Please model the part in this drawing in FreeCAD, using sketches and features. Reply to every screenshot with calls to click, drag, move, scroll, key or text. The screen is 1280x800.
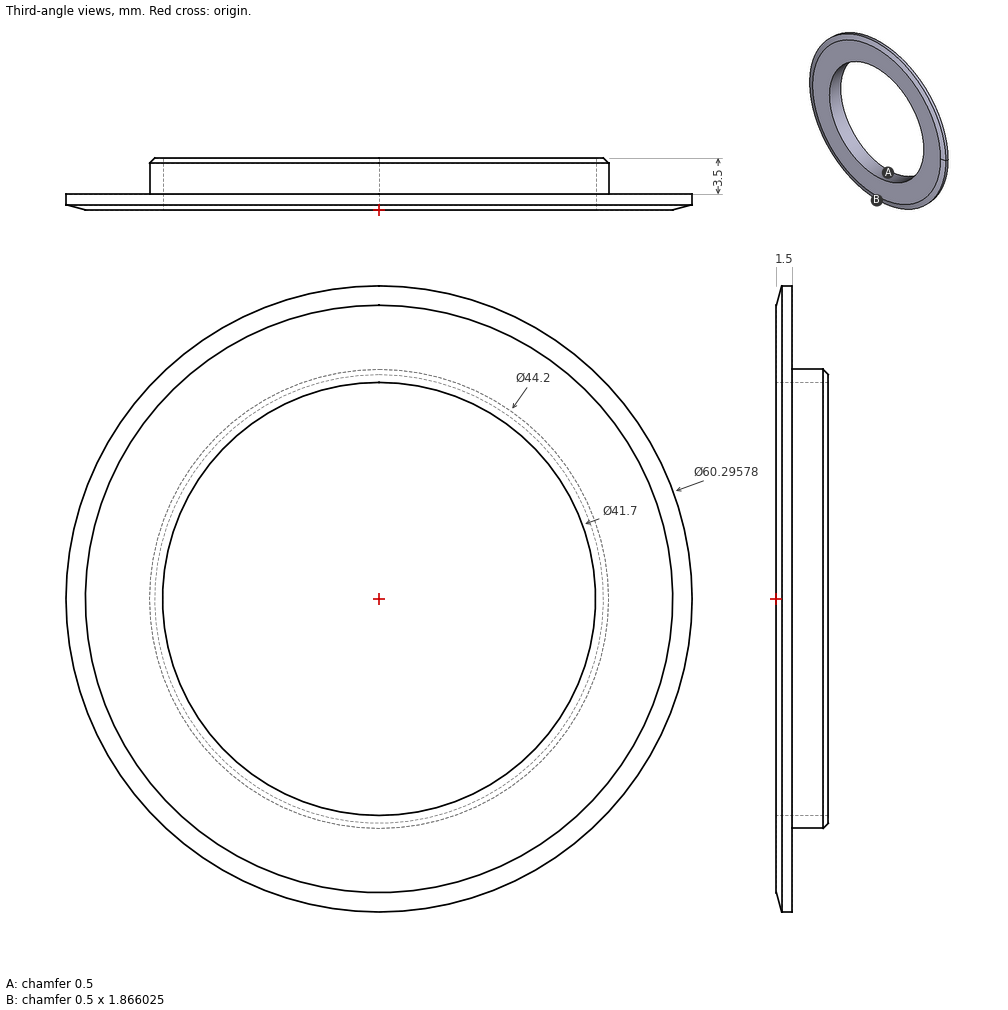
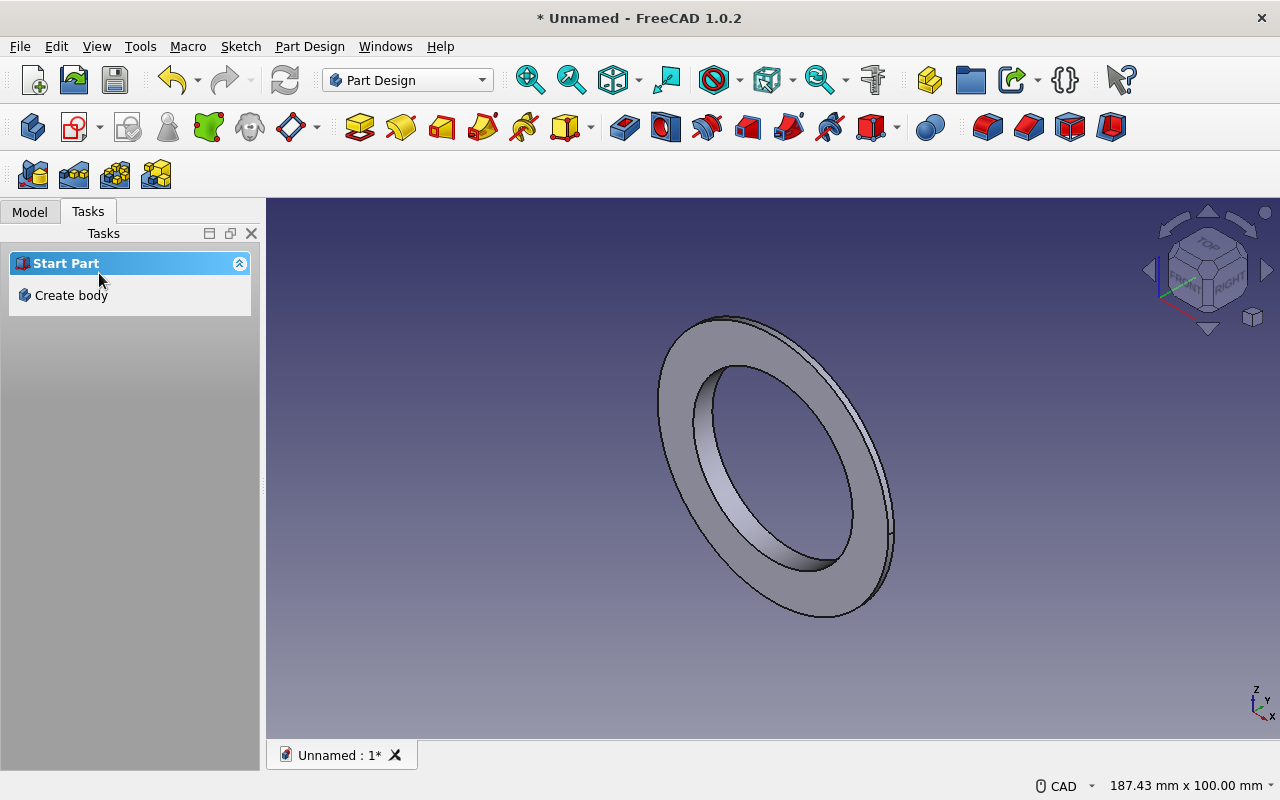
click(737, 320)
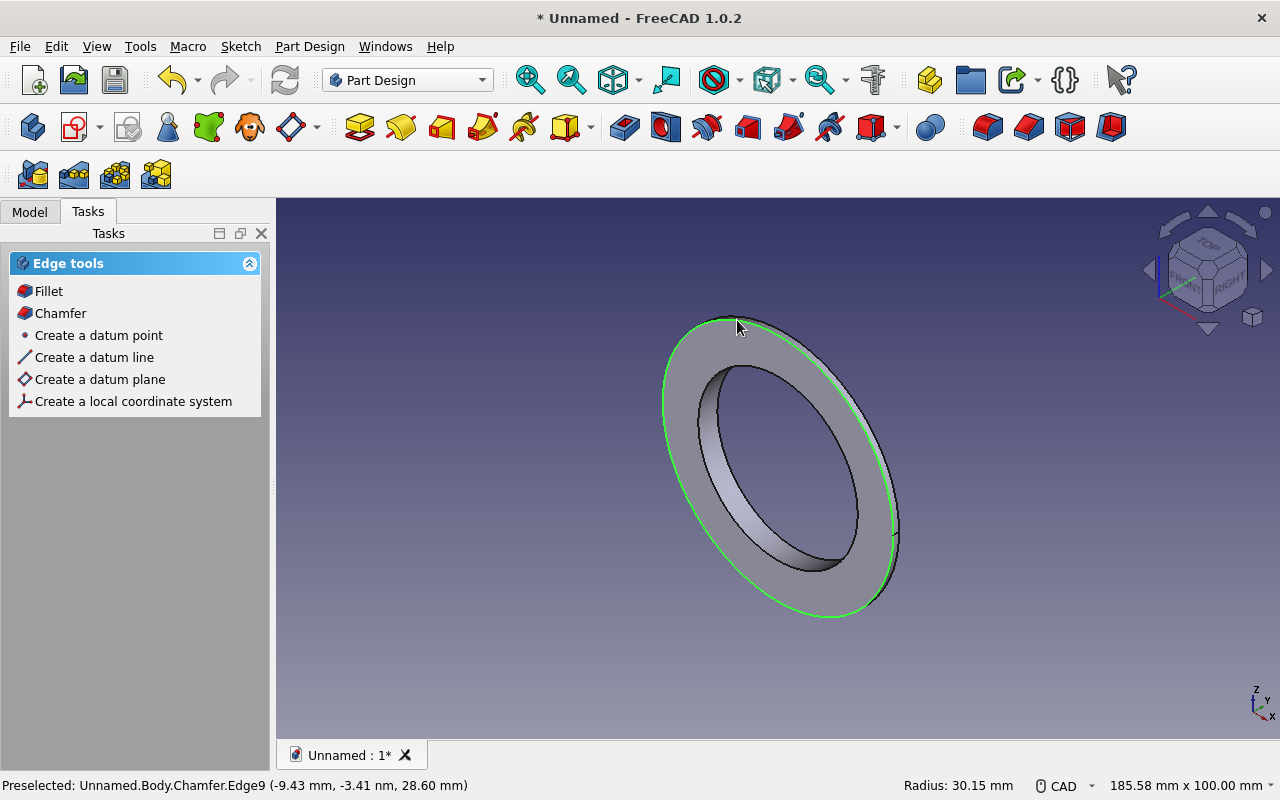
click(1029, 128)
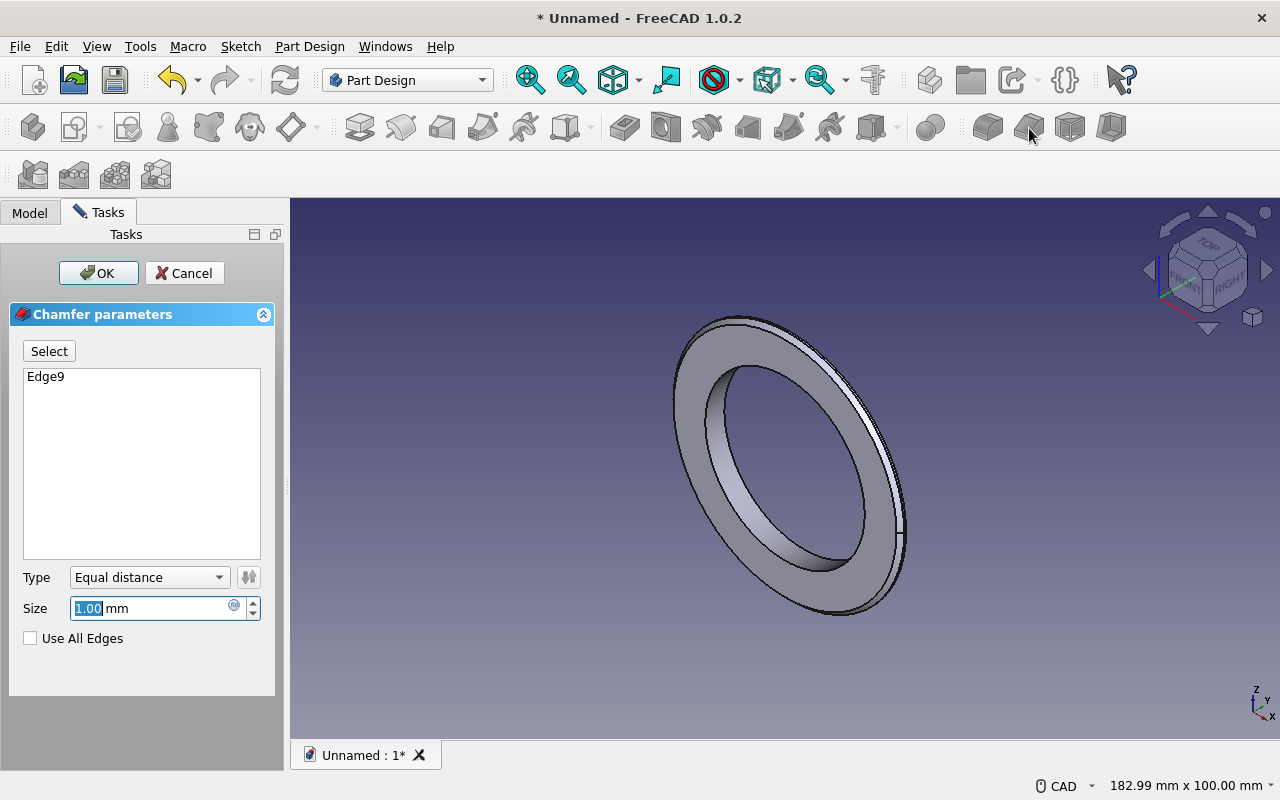
text(0.5)
key(Tab)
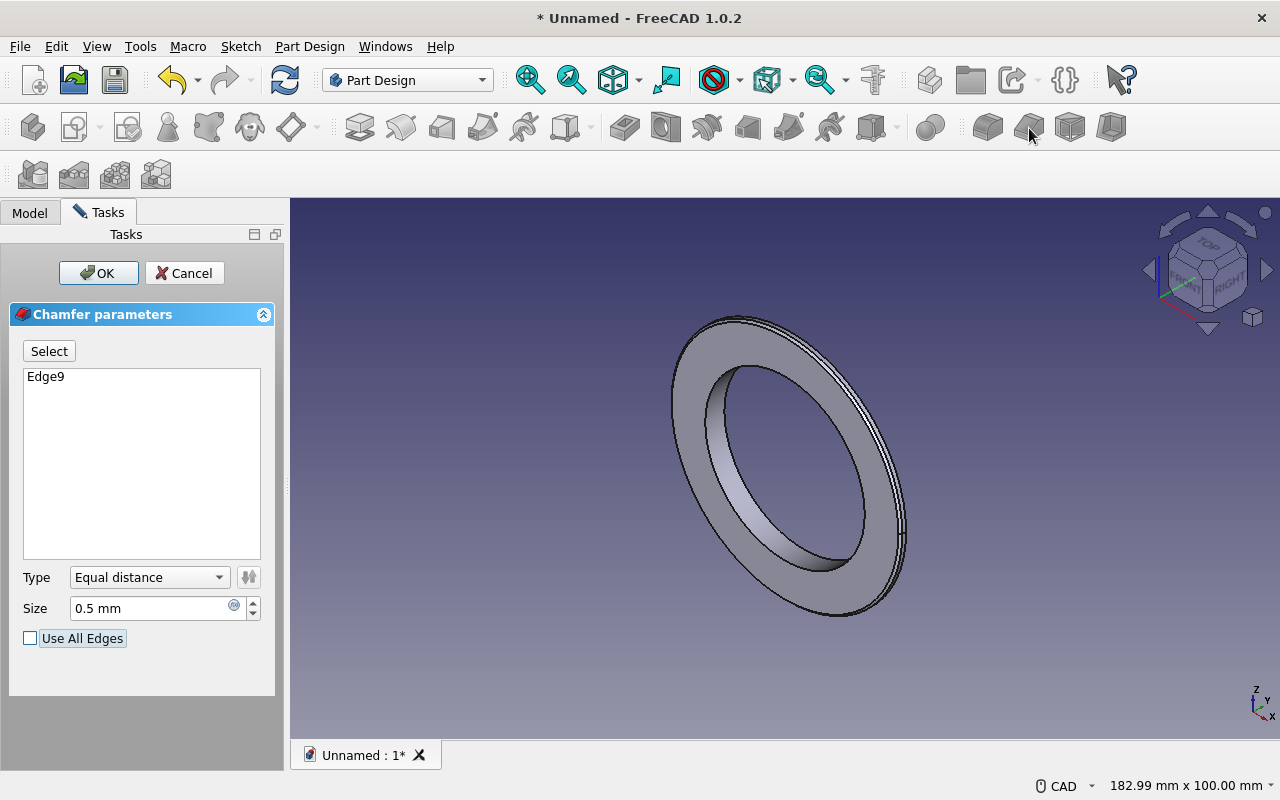
click(150, 578)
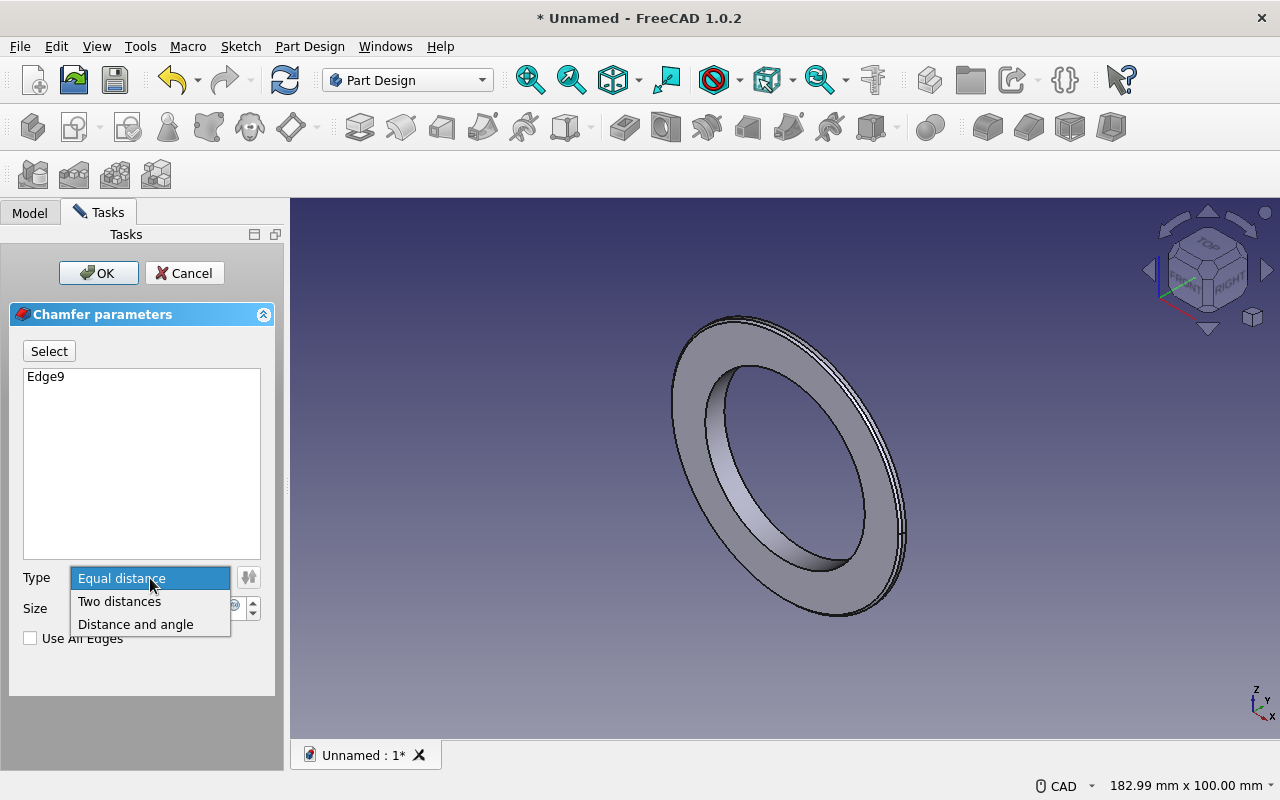
click(148, 602)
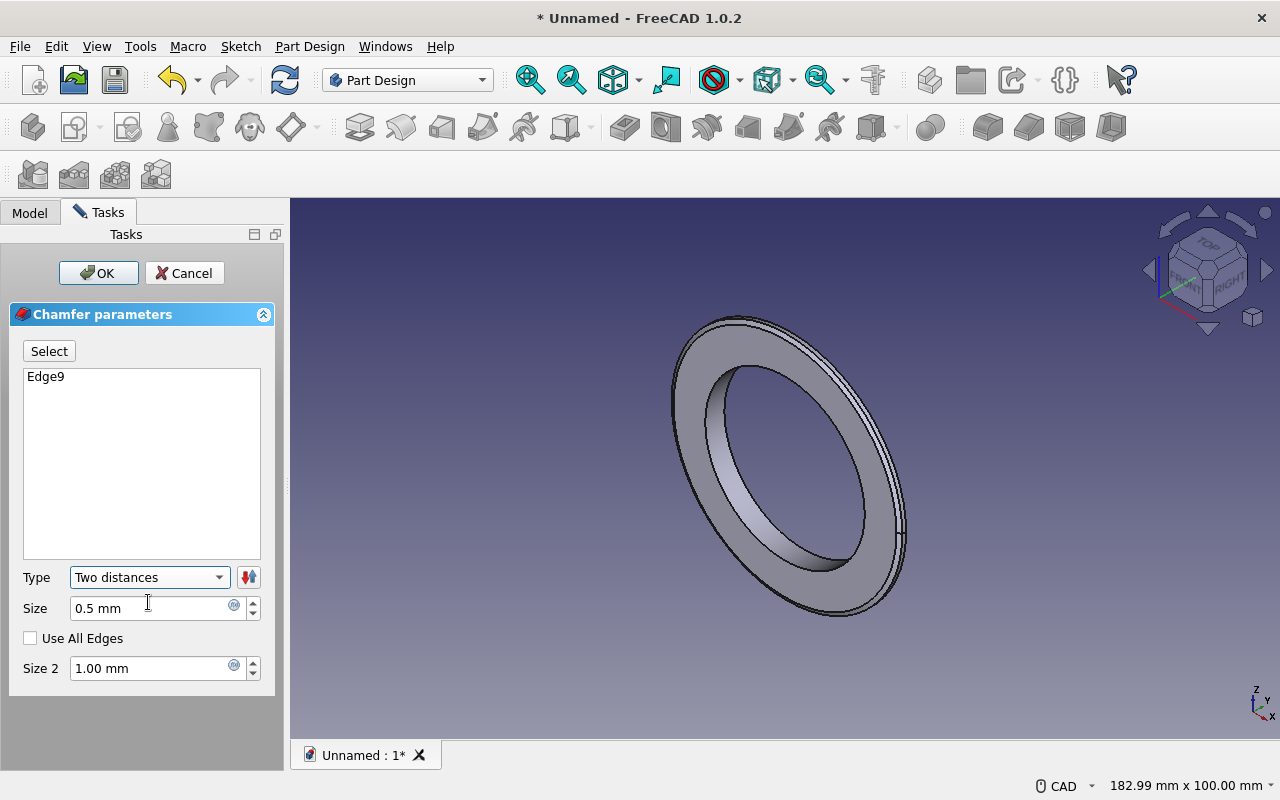
triple_click(158, 668)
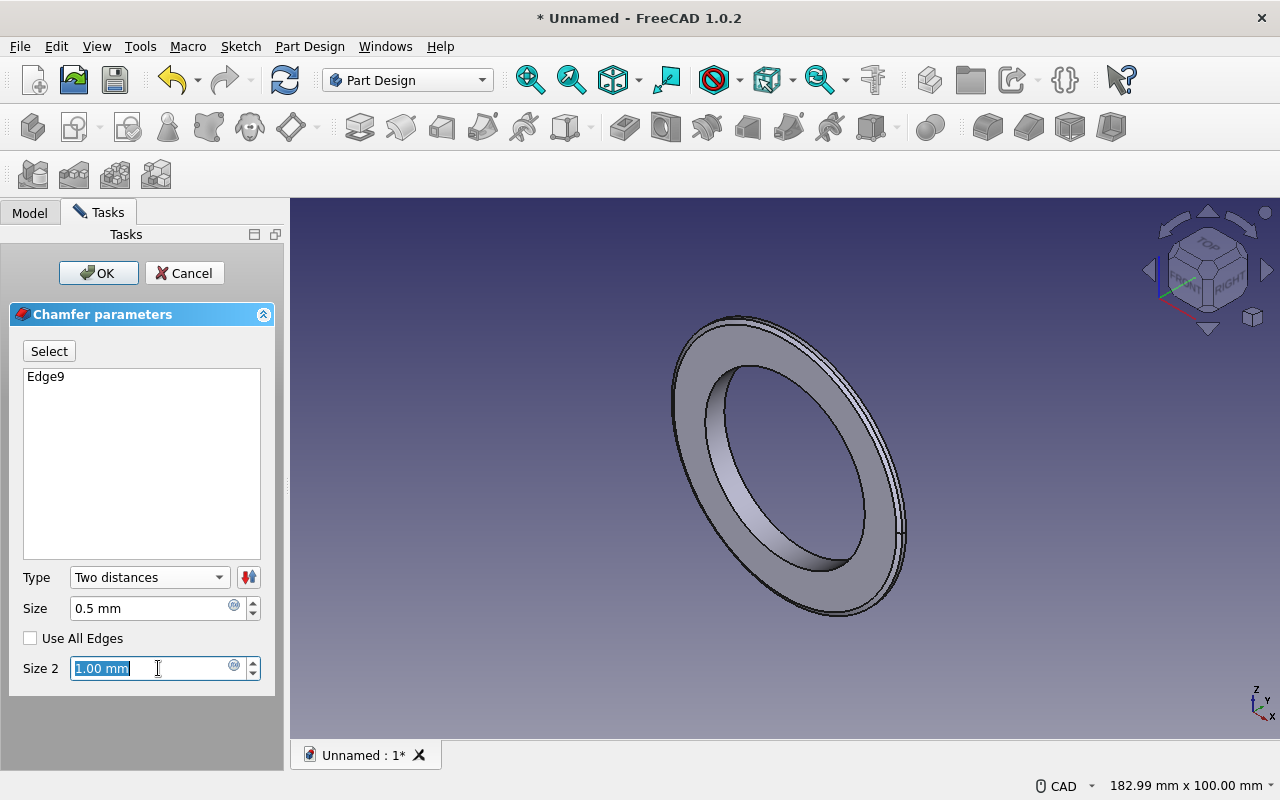
text(1.866025)
key(Tab)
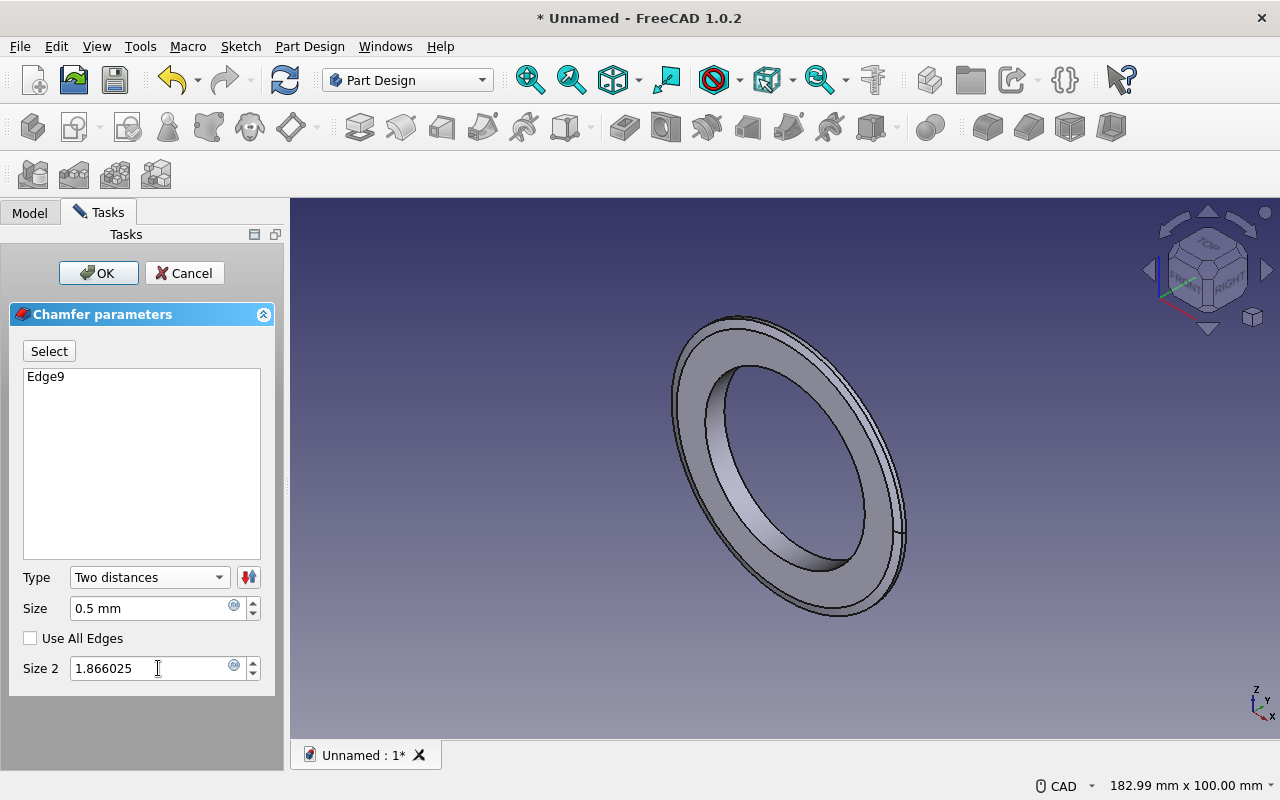
click(99, 273)